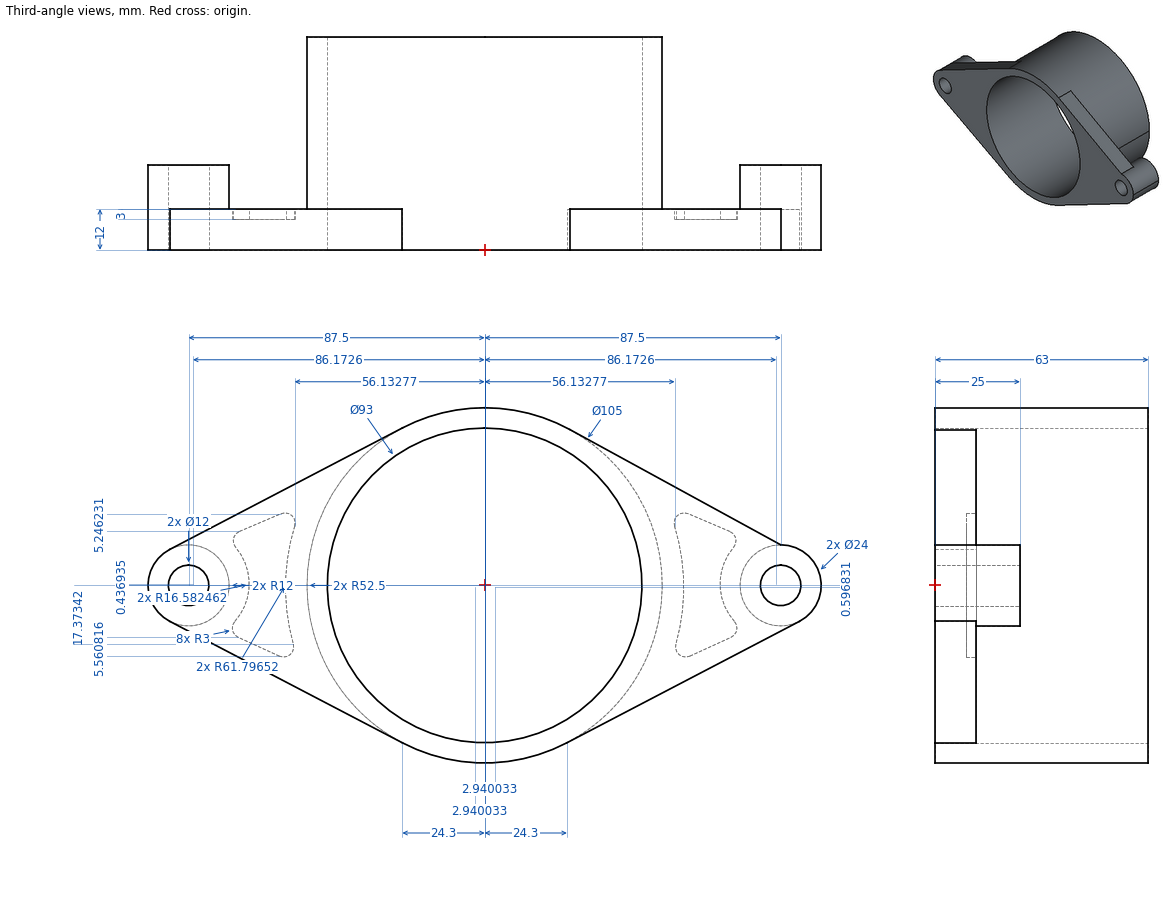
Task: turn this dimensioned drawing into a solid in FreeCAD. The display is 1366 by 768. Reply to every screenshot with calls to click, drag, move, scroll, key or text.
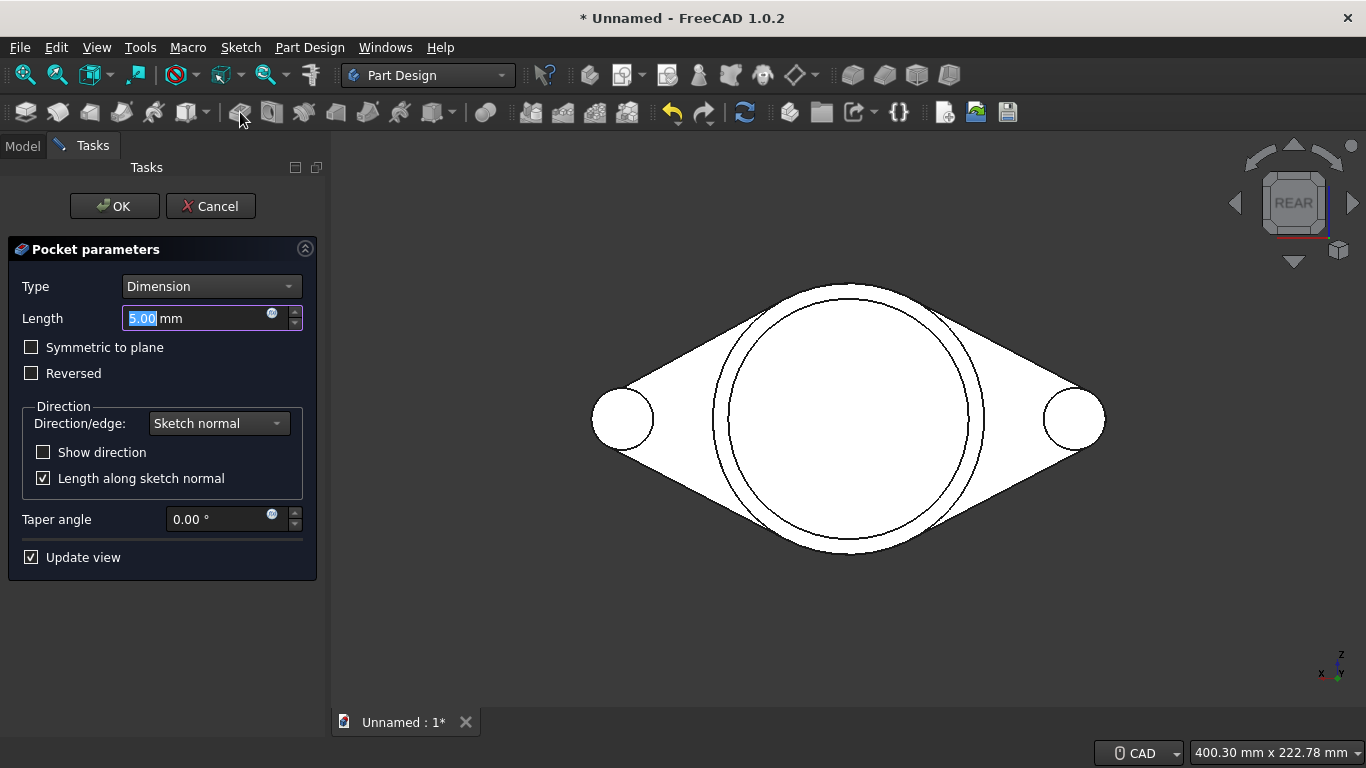
click(212, 286)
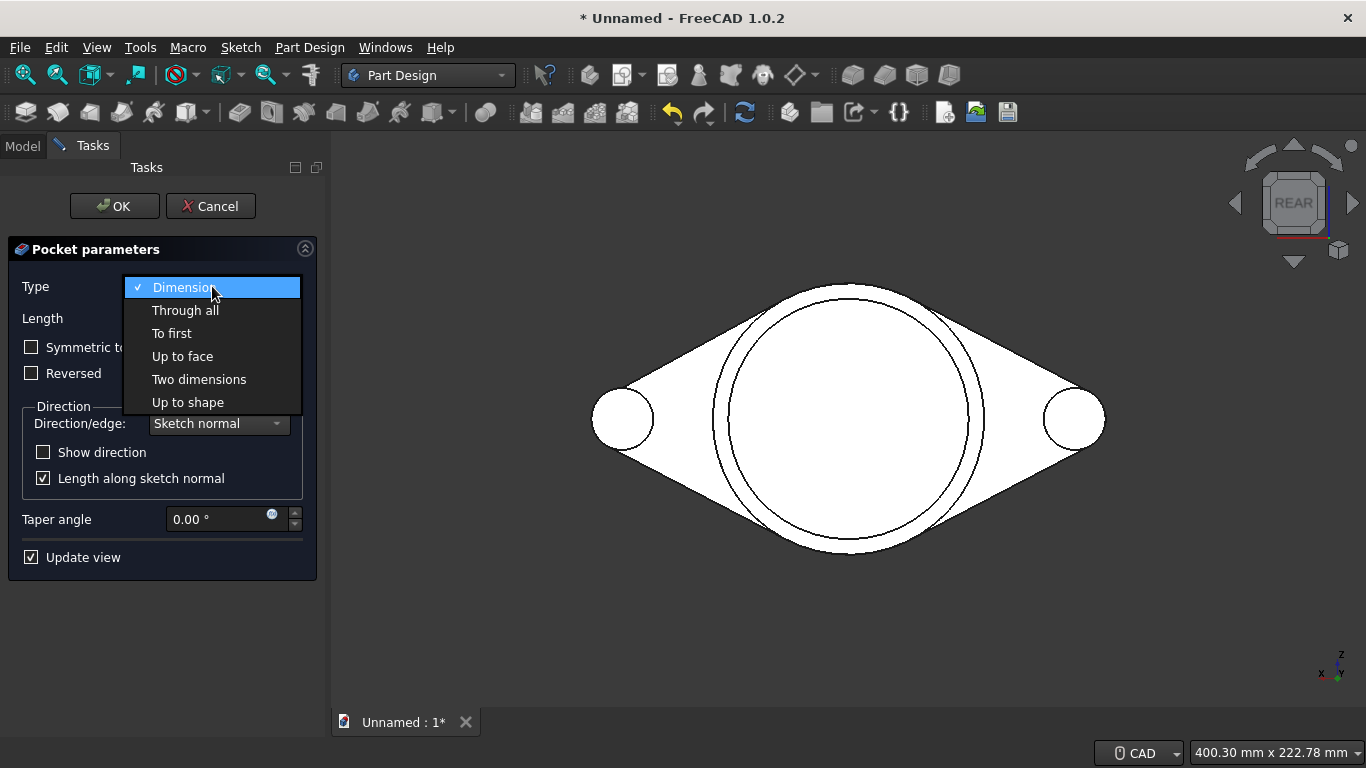
click(212, 310)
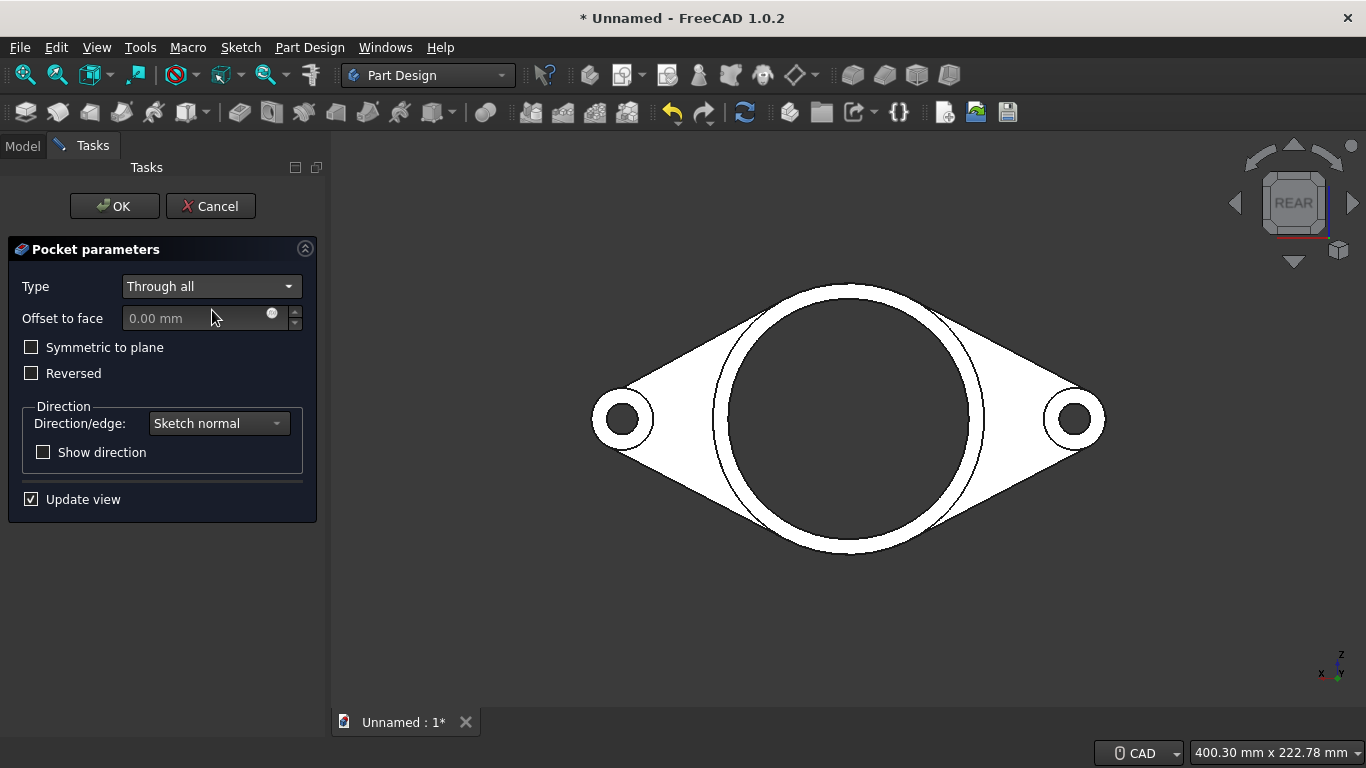
click(115, 206)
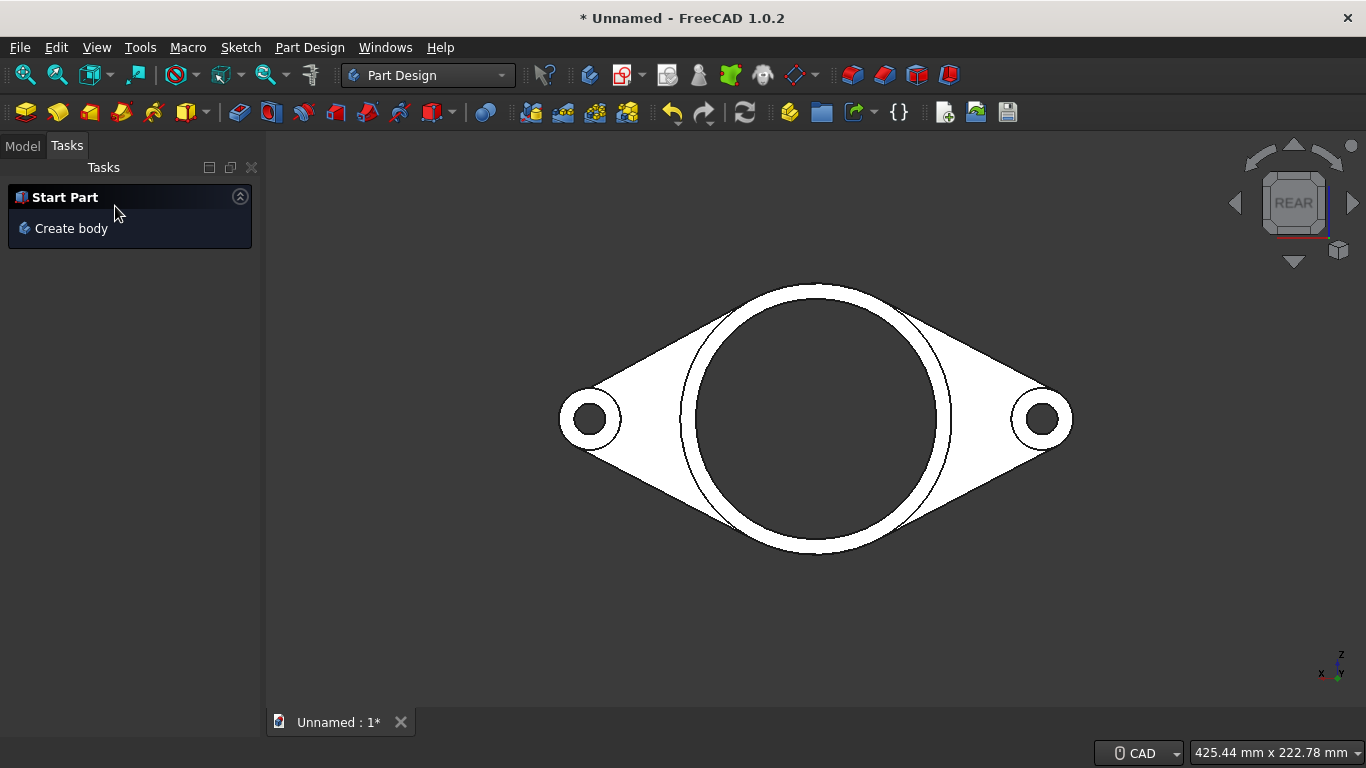
click(993, 452)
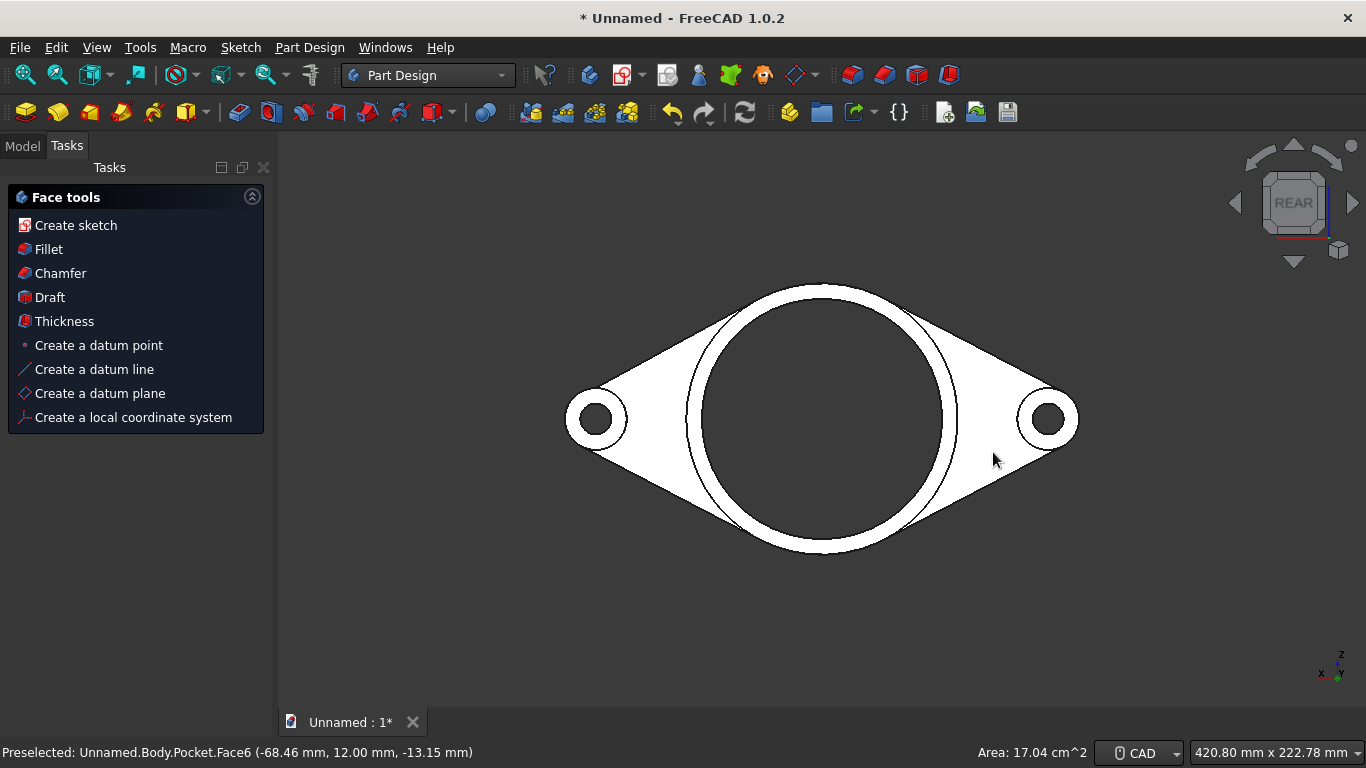
click(622, 76)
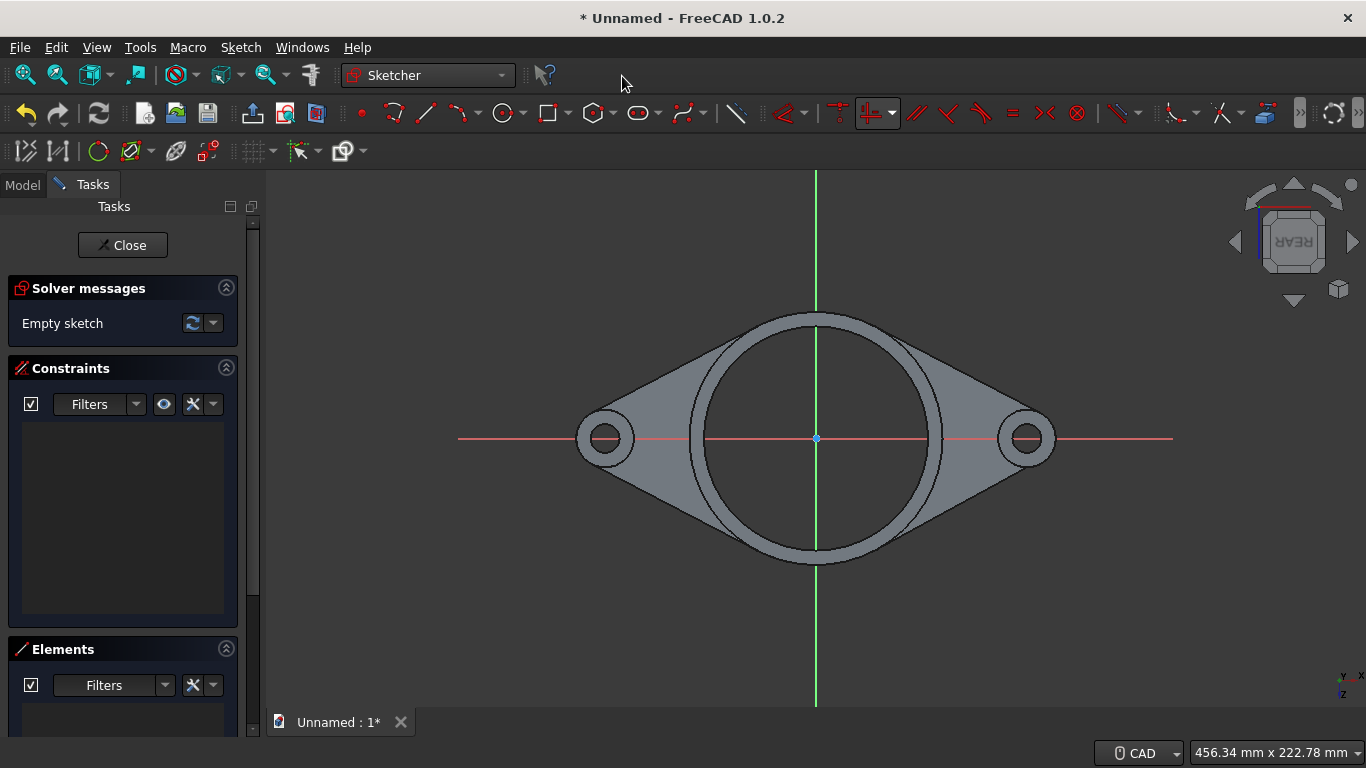
click(318, 114)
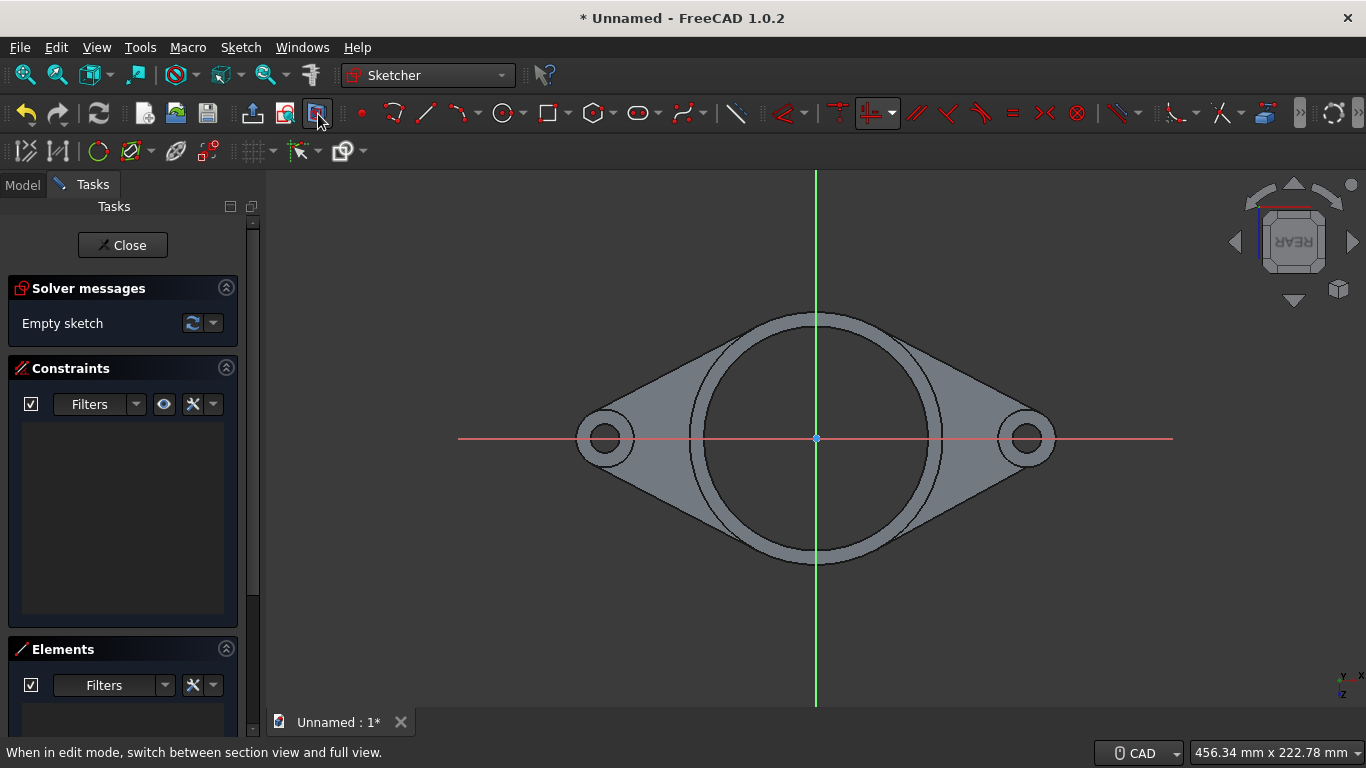
scroll(899, 439, up, 3)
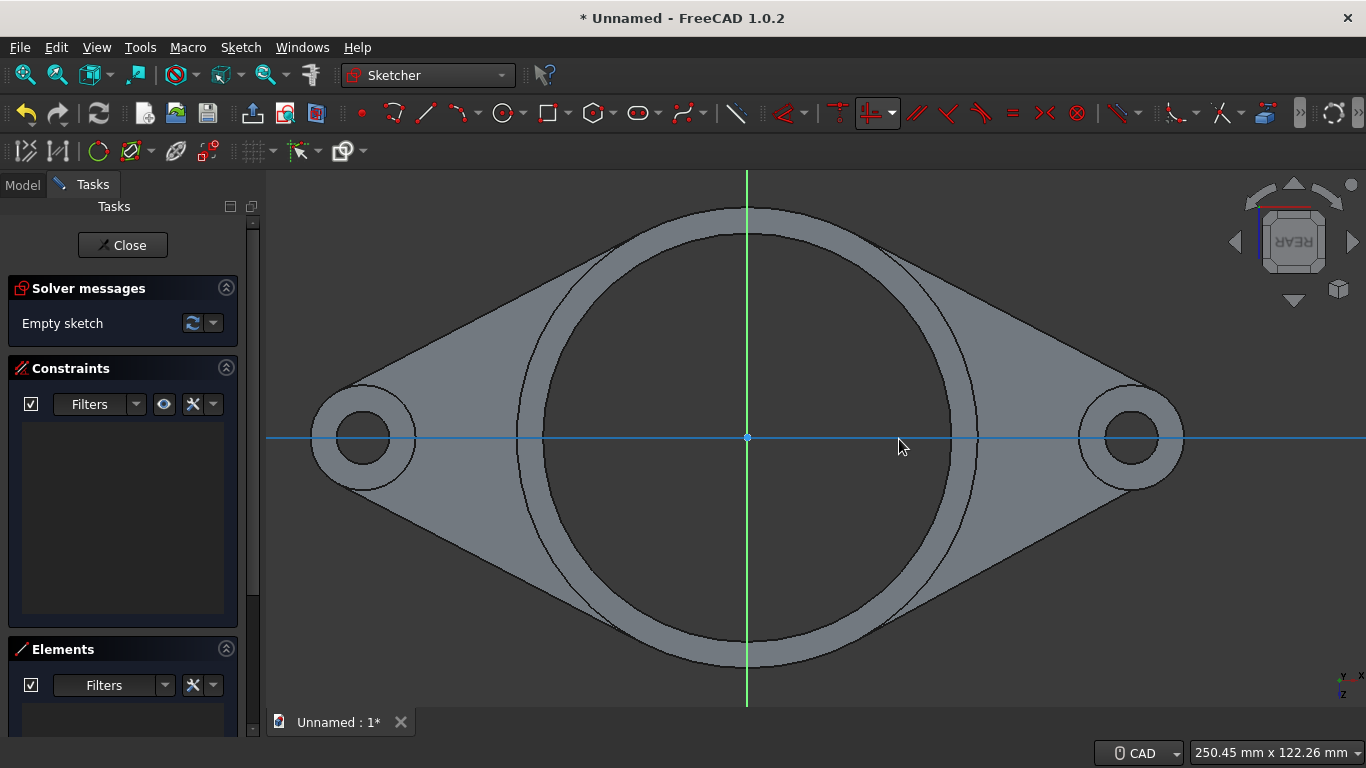
key(g)
key(l)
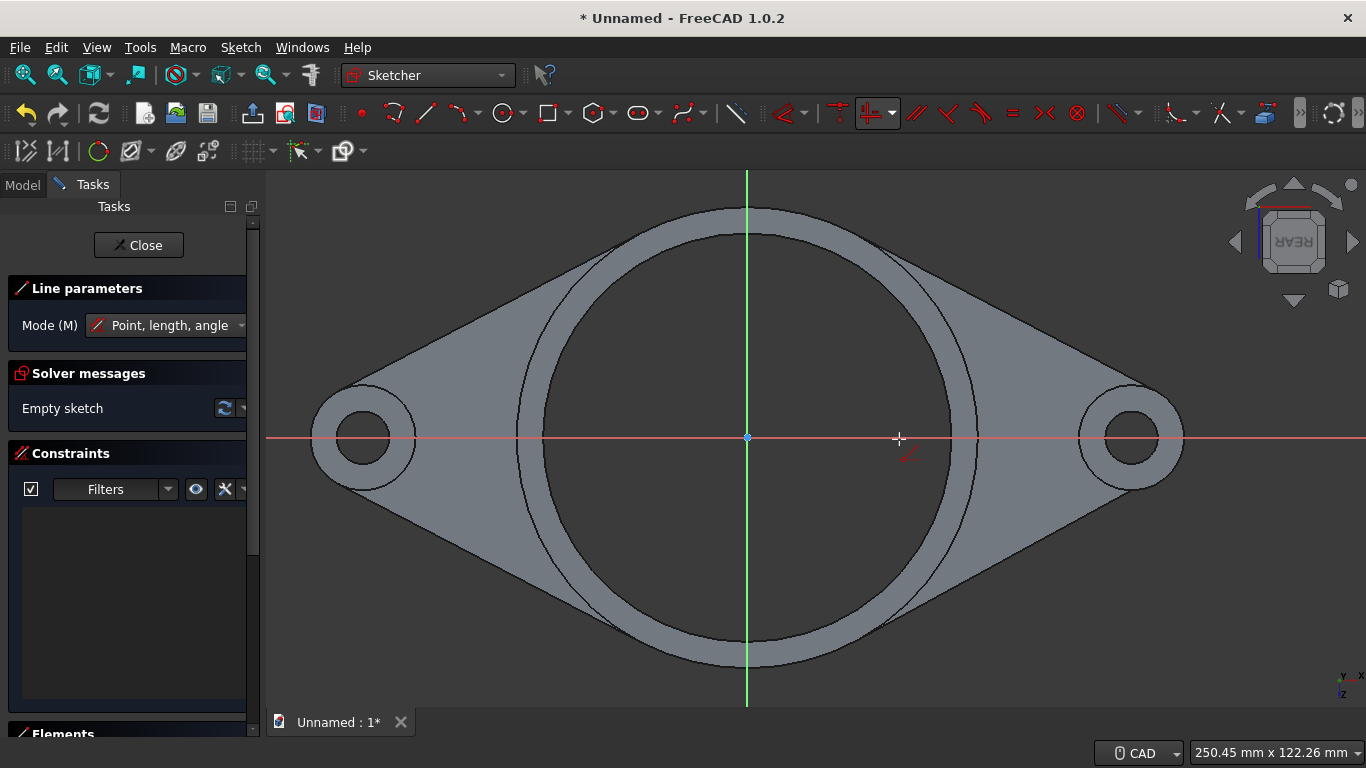
click(481, 346)
click(427, 370)